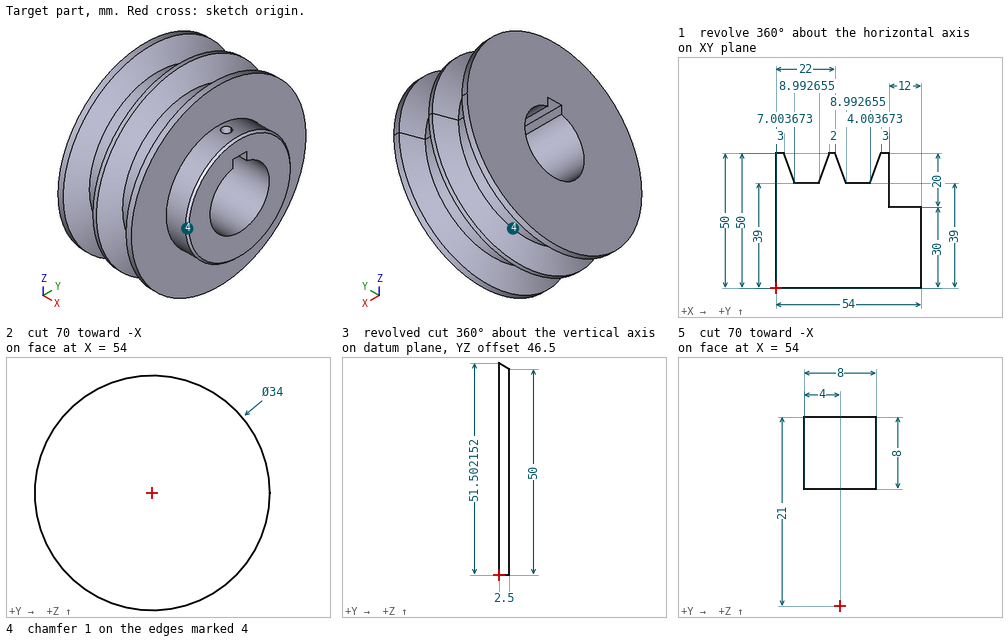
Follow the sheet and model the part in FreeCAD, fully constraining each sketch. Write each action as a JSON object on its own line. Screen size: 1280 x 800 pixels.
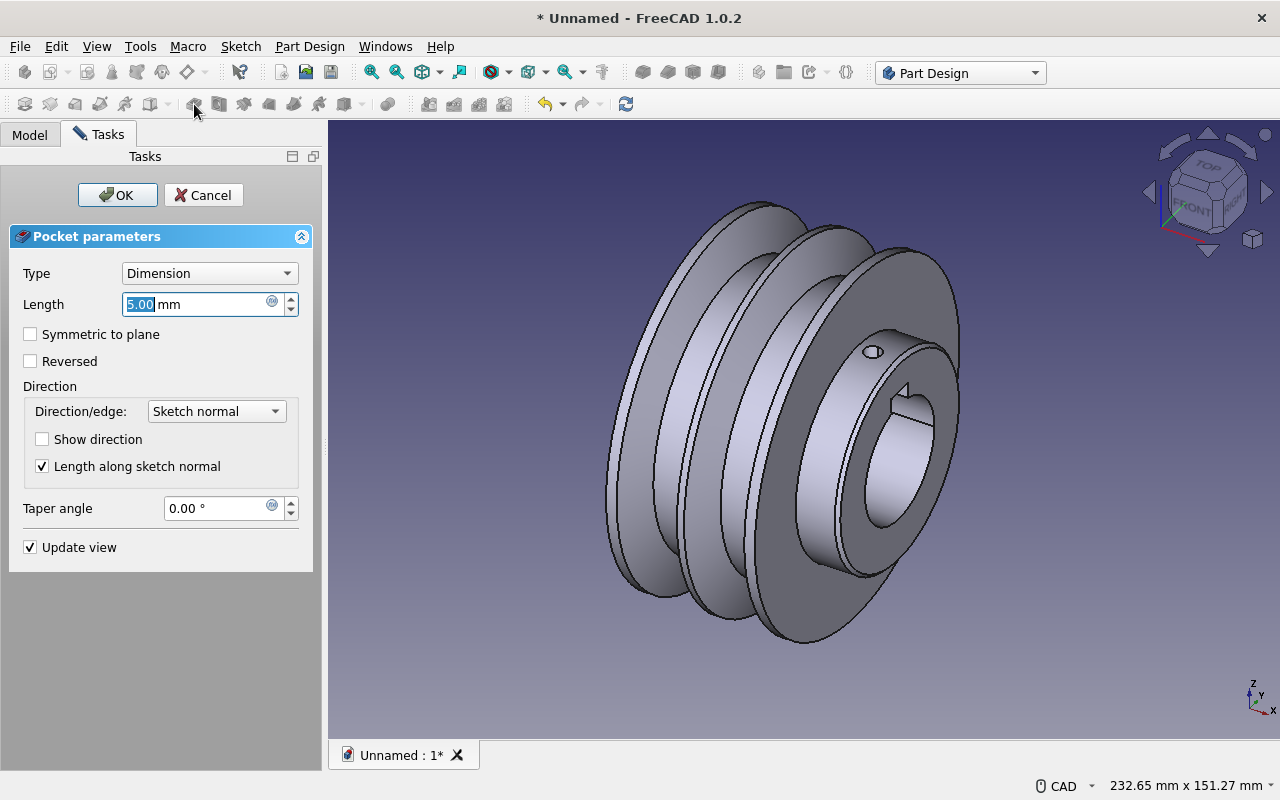
{"action": "type", "text": "70"}
{"action": "key", "text": "Tab"}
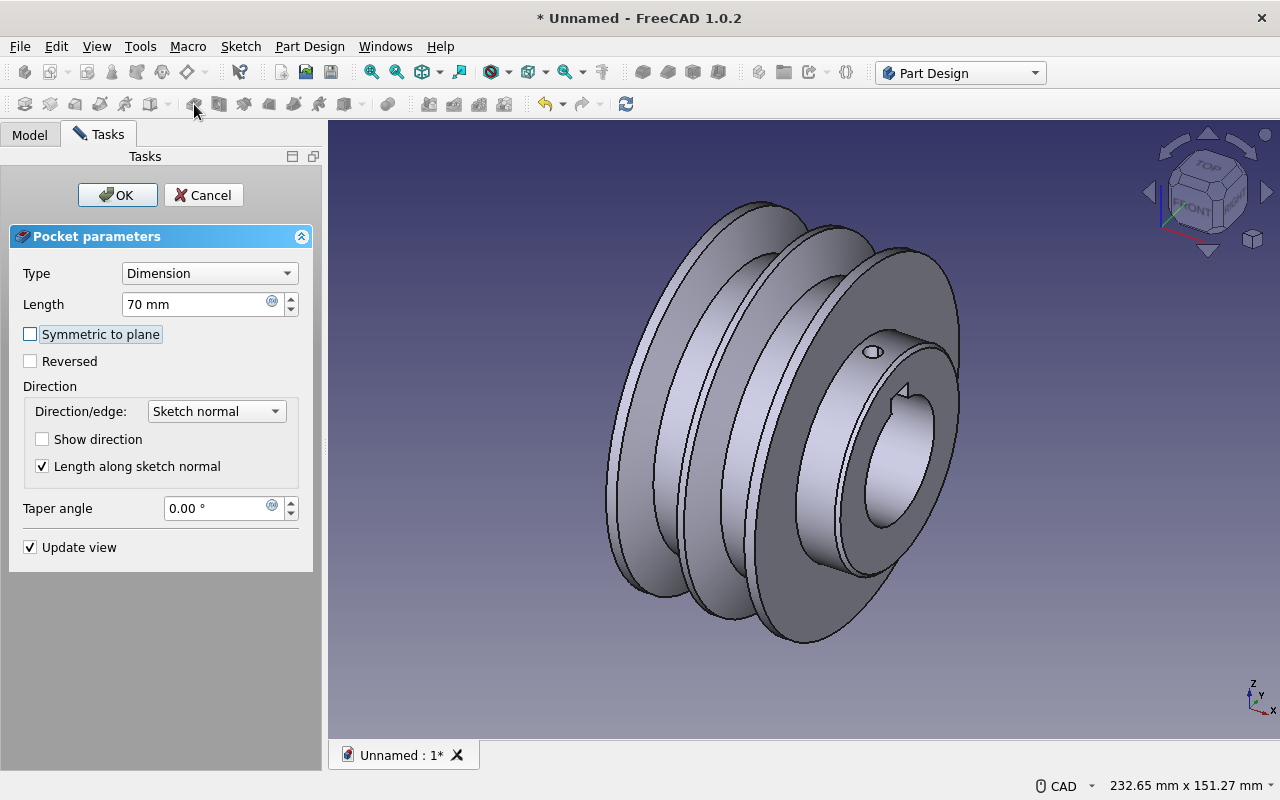
{"action": "left_click", "coordinate": [118, 195]}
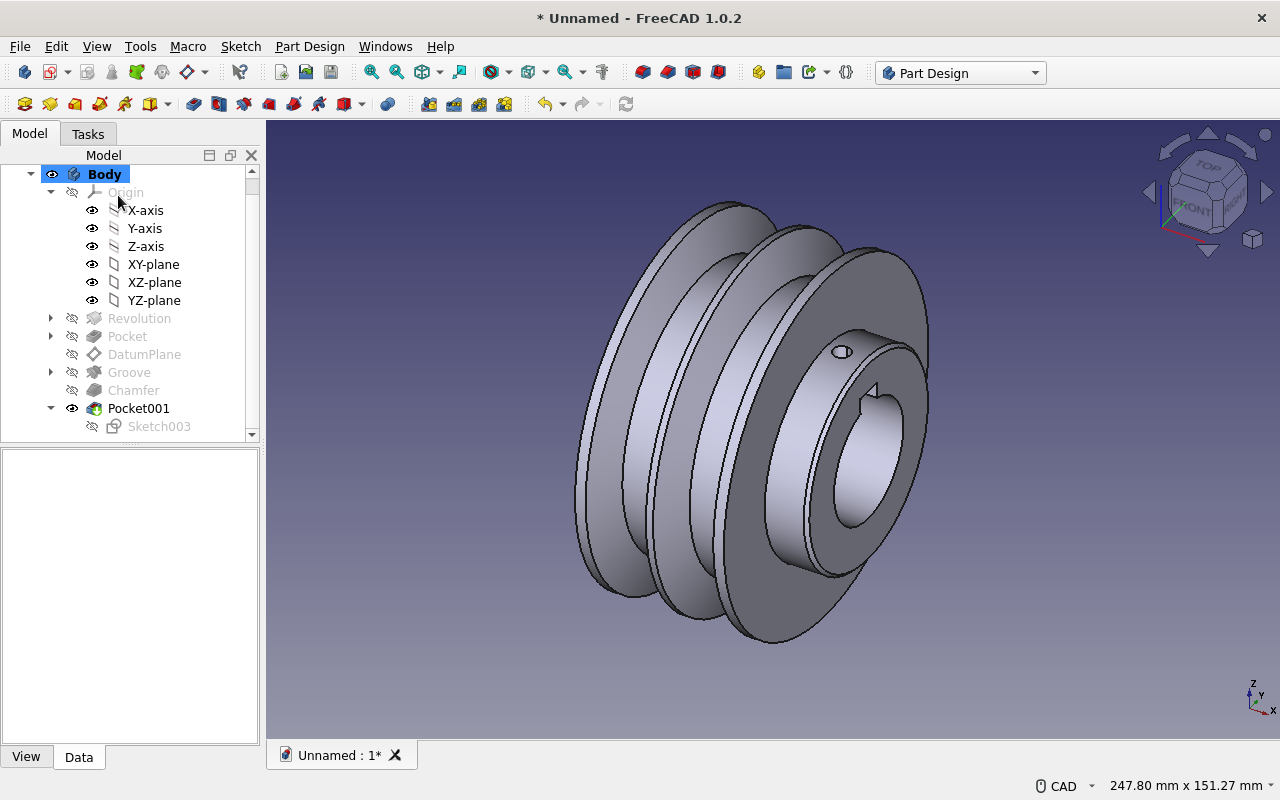
{"action": "key", "text": "0"}